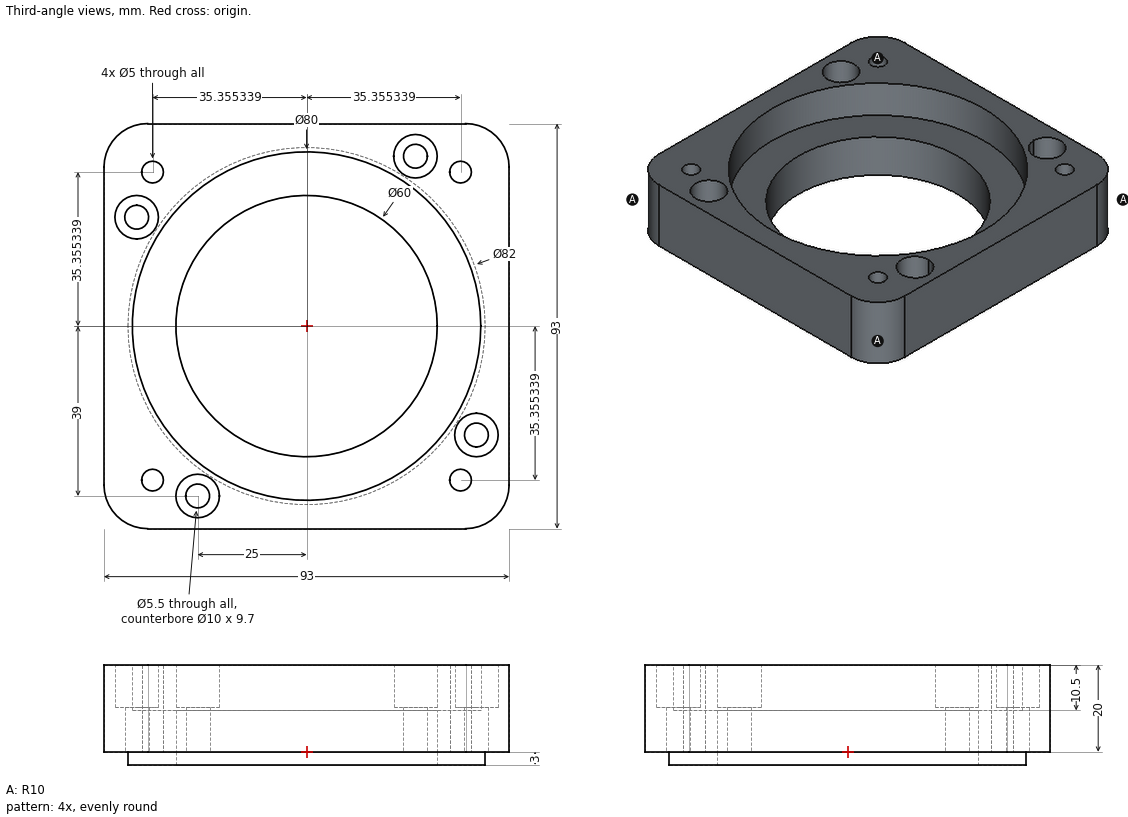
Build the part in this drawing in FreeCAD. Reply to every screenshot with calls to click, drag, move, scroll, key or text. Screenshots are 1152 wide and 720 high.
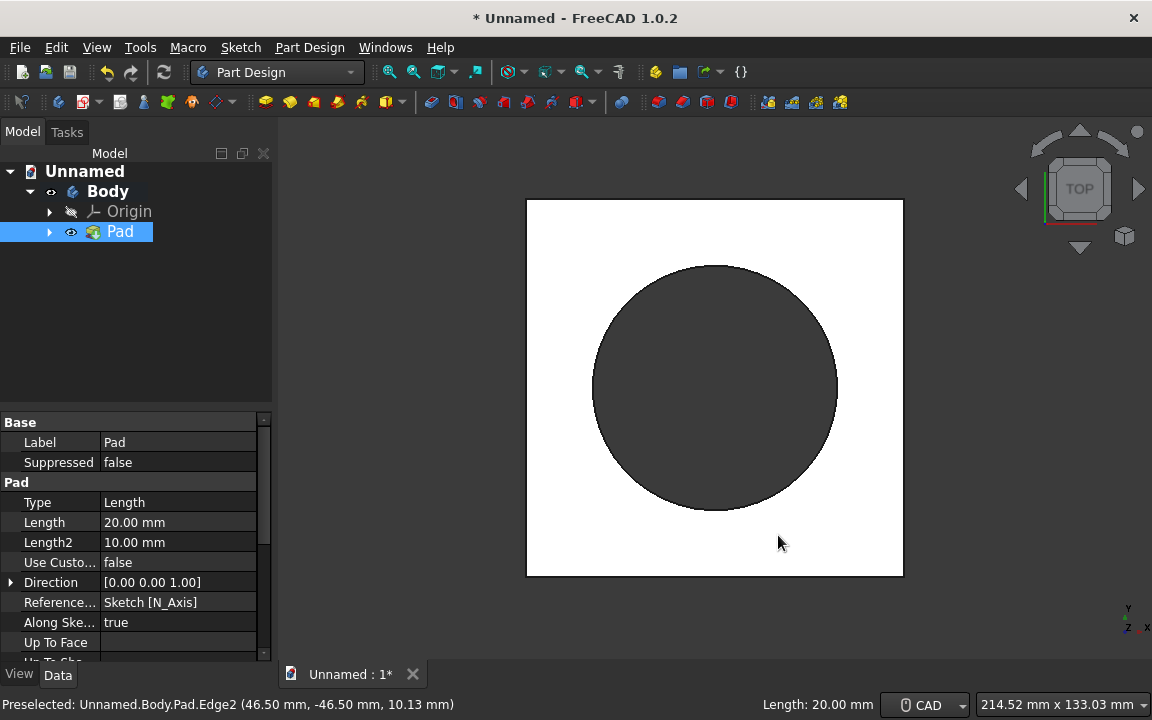
key(1)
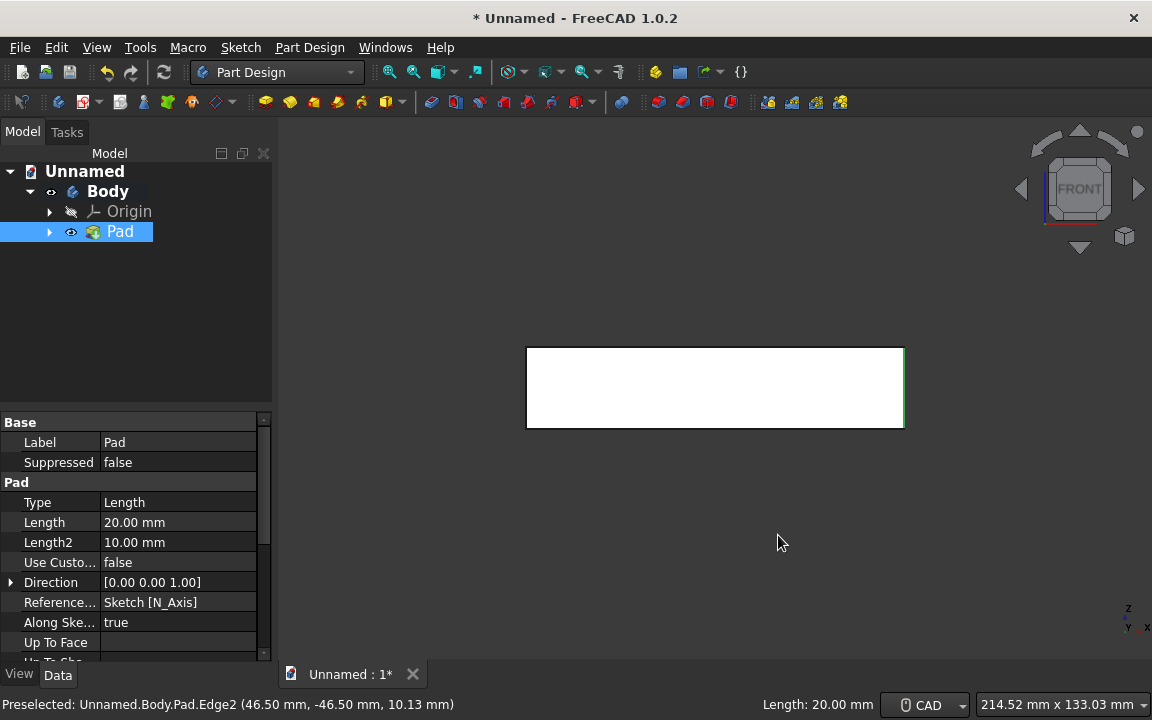
click(390, 72)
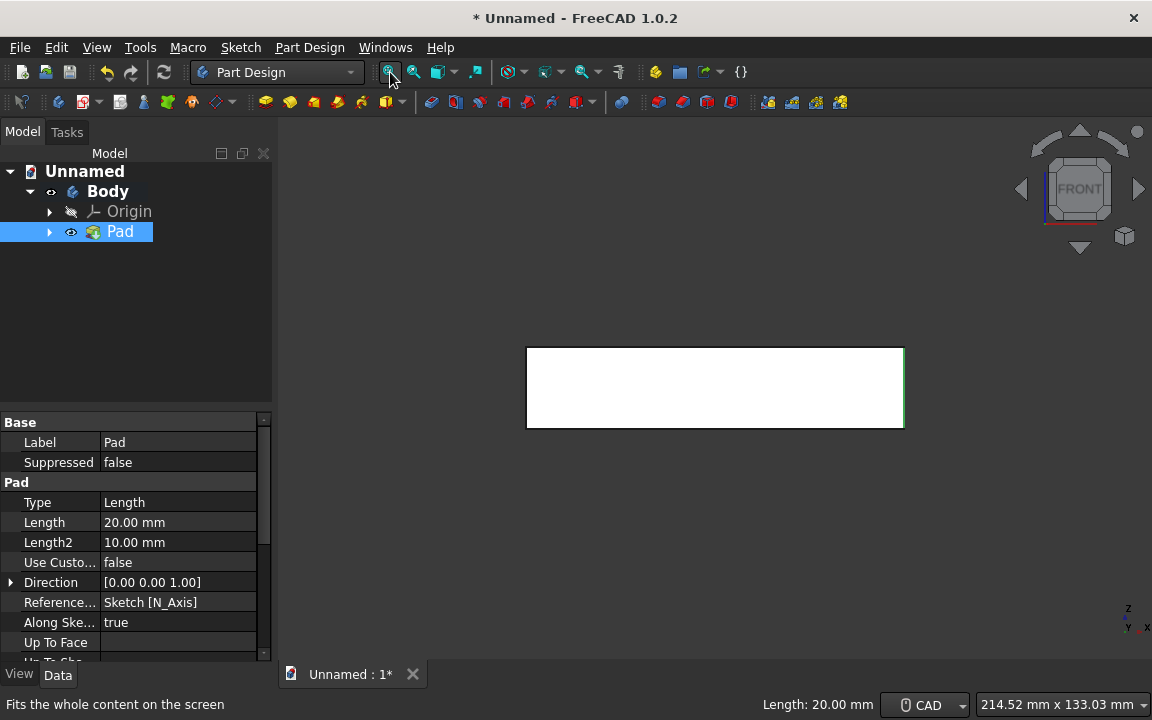
click(526, 387, ctrl)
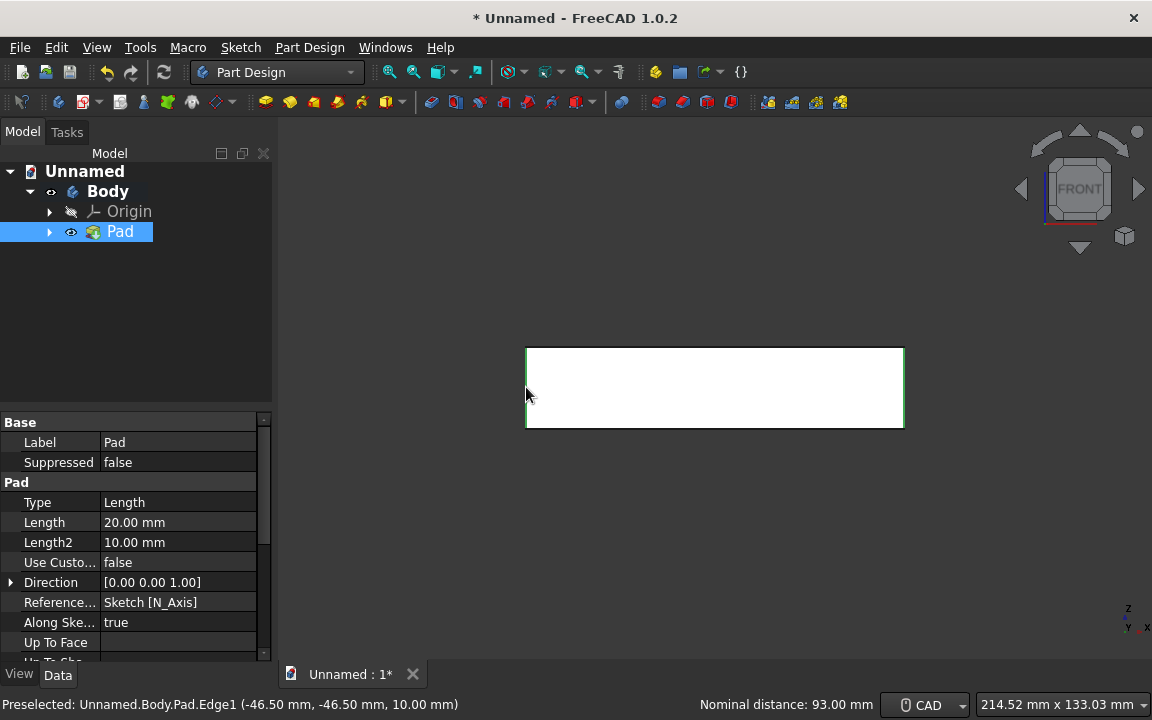
key(3)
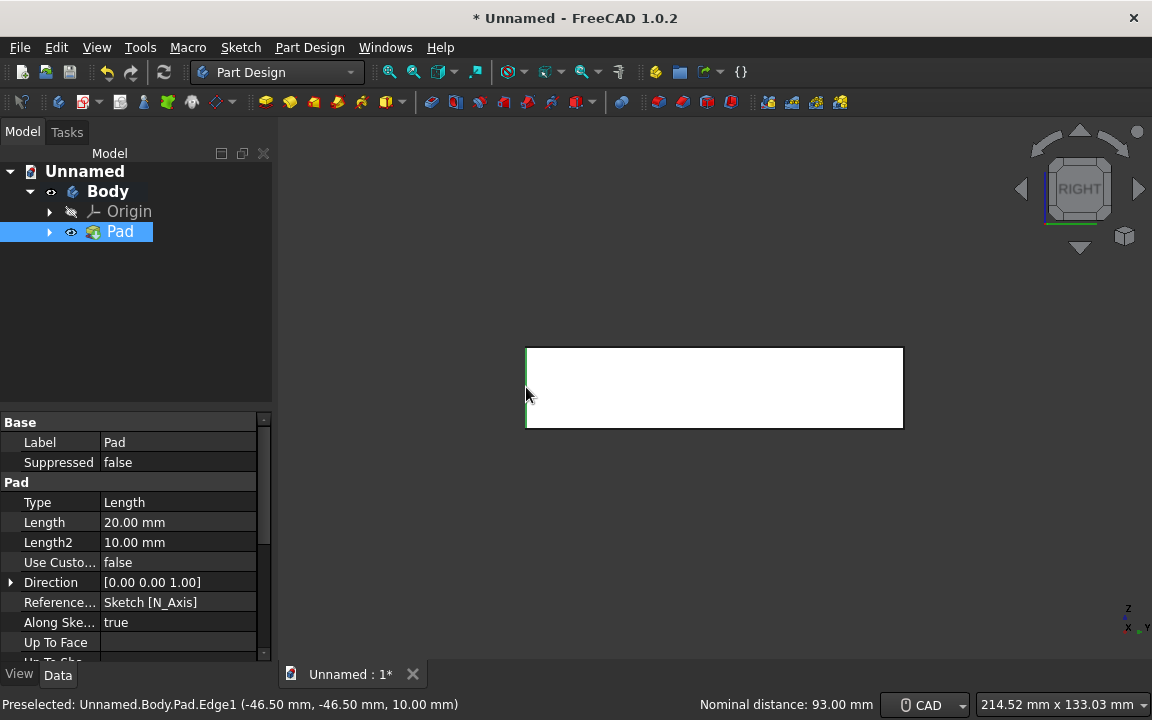
click(390, 72)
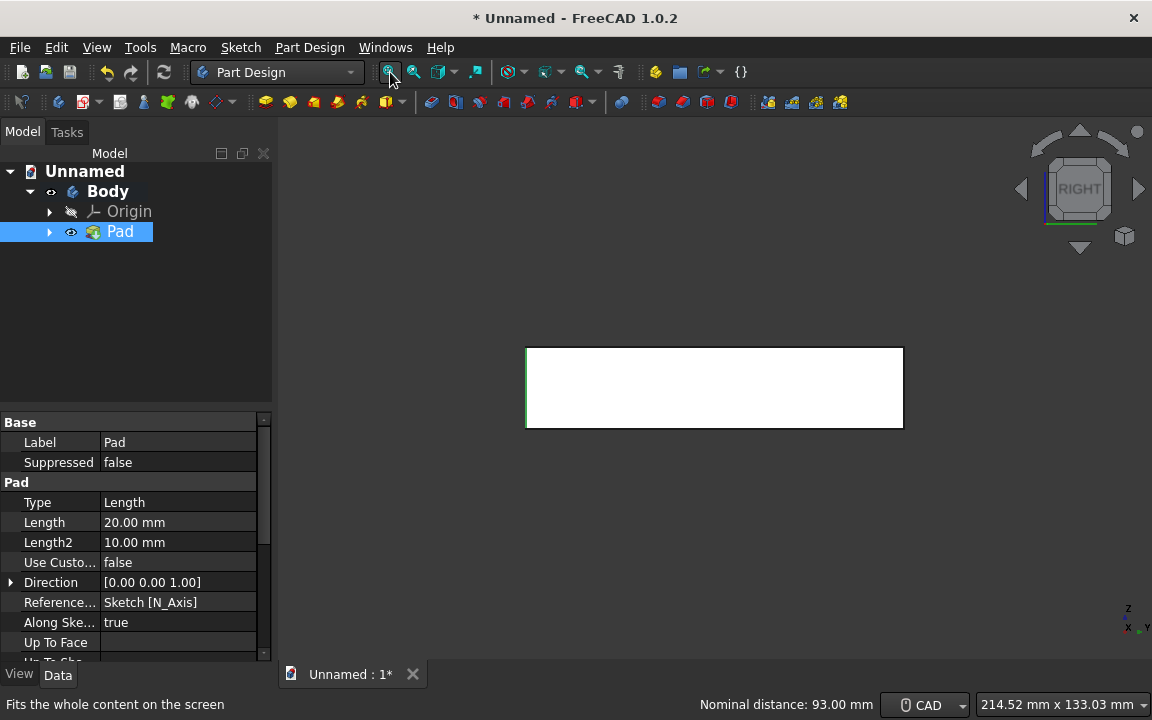
click(904, 387, ctrl)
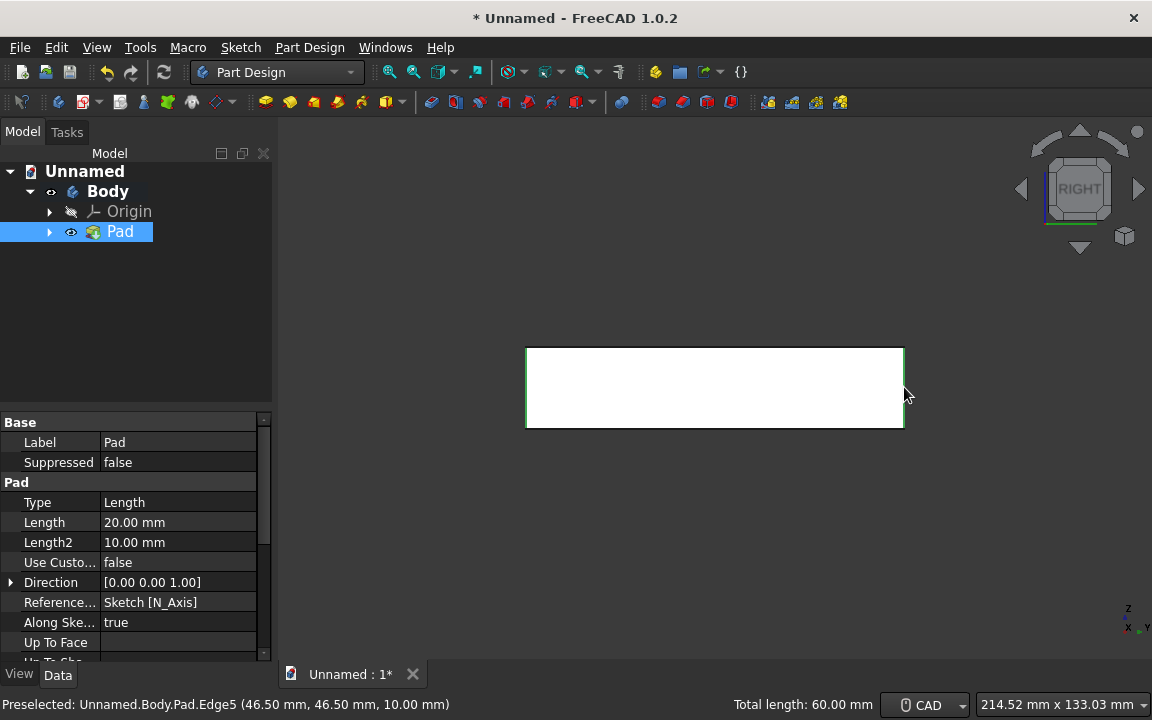
key(5)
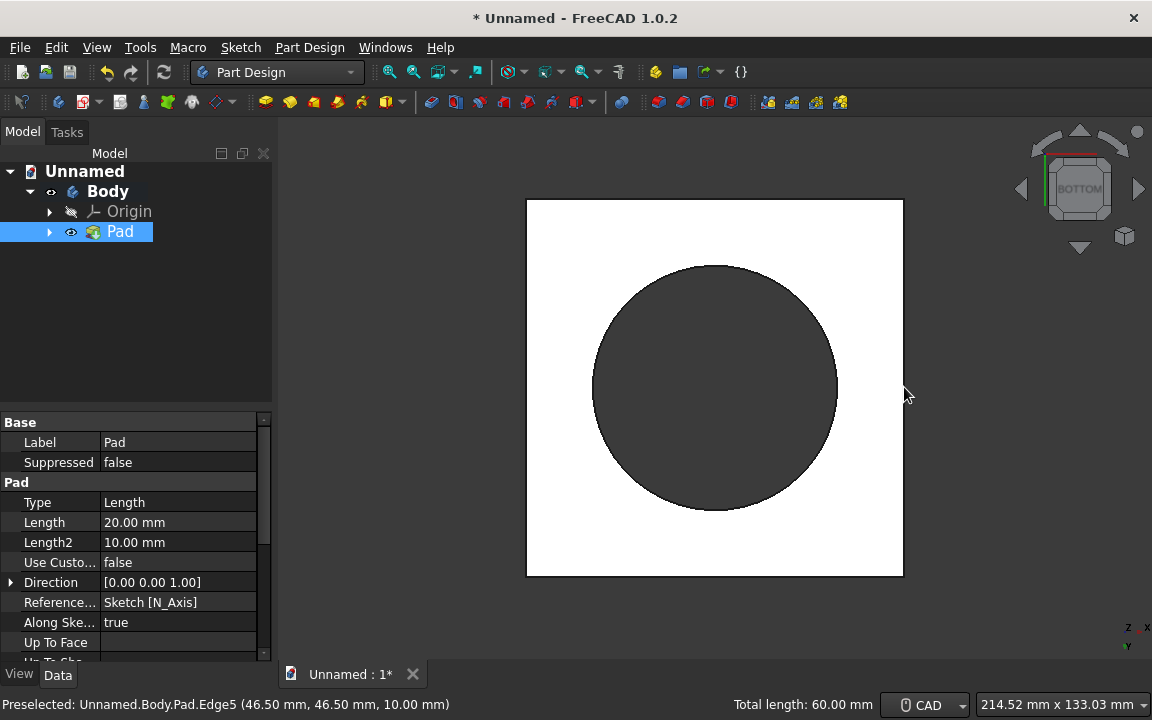
key(4)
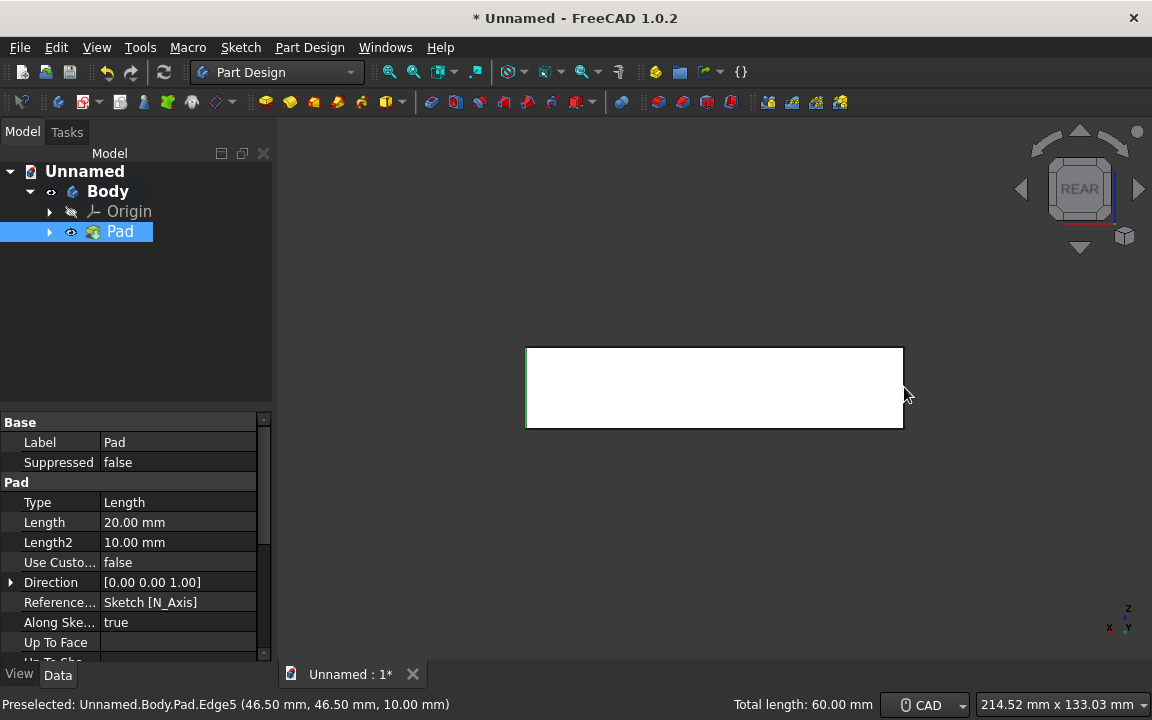
click(390, 72)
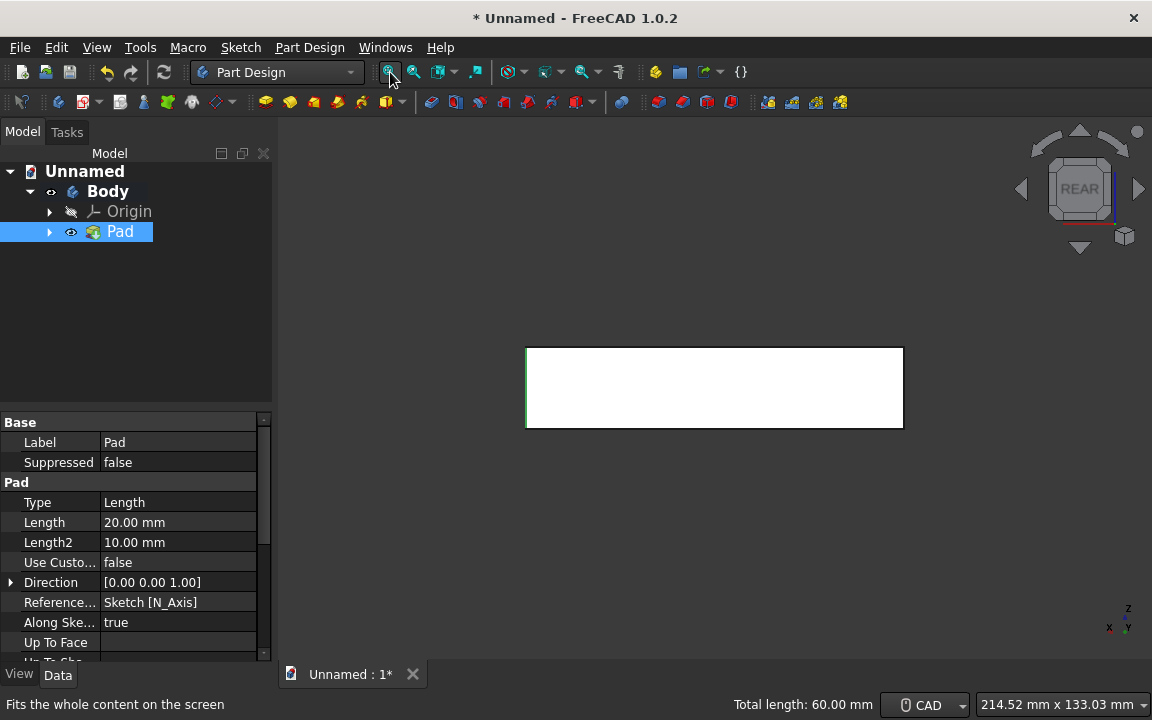
click(904, 387, ctrl)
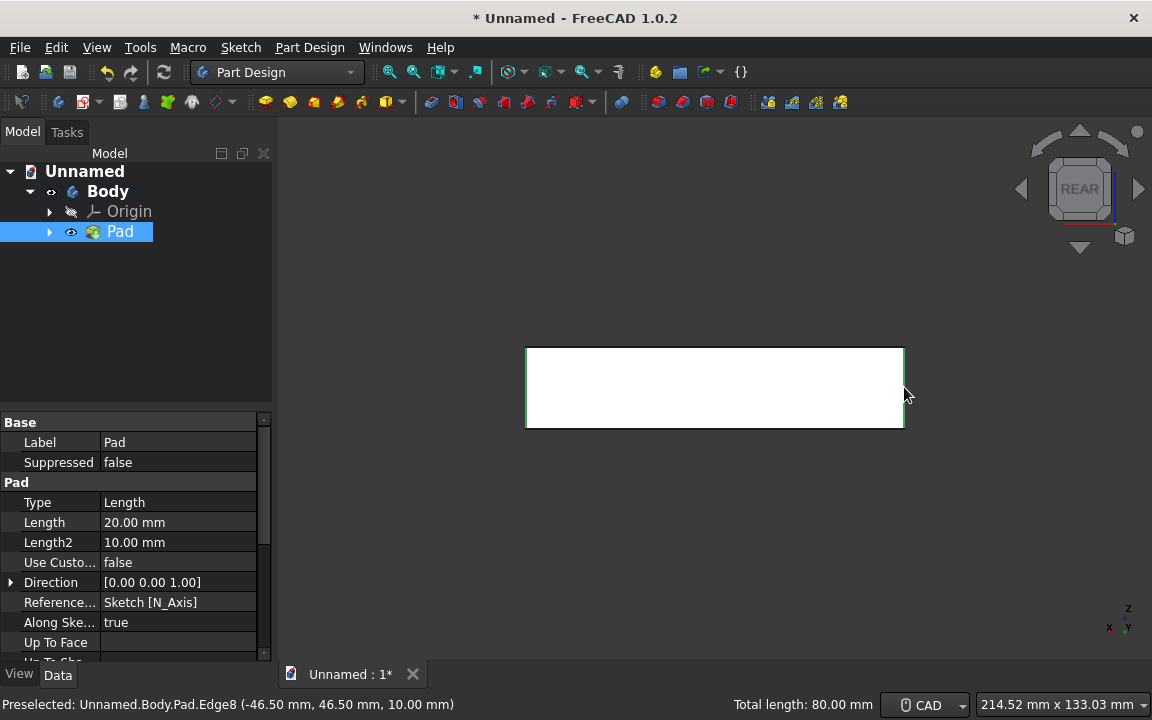
click(660, 102)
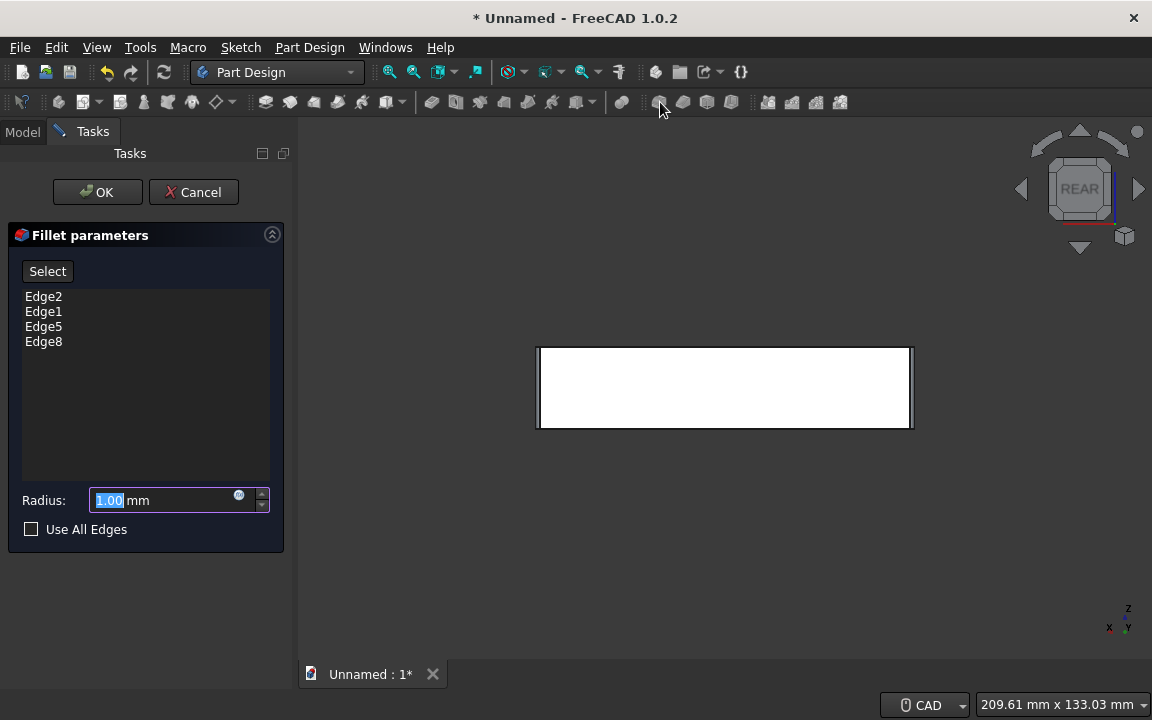
text(10)
key(Tab)